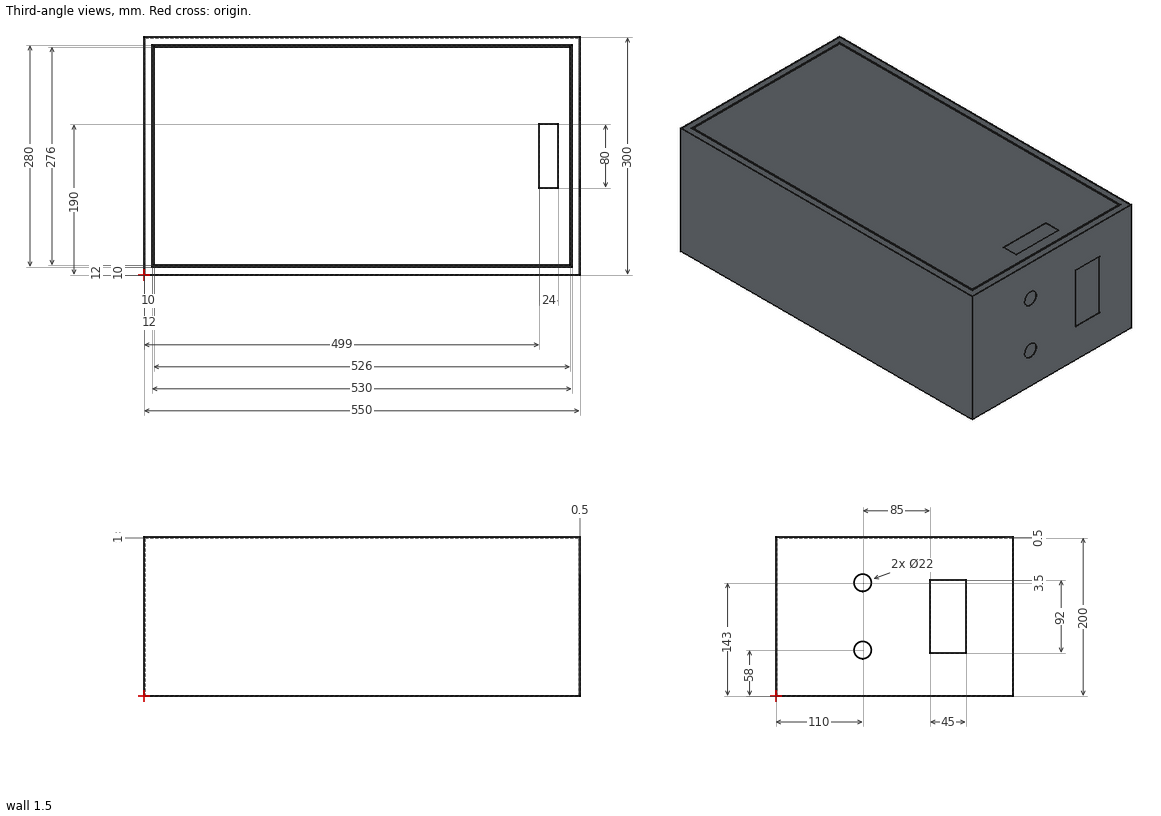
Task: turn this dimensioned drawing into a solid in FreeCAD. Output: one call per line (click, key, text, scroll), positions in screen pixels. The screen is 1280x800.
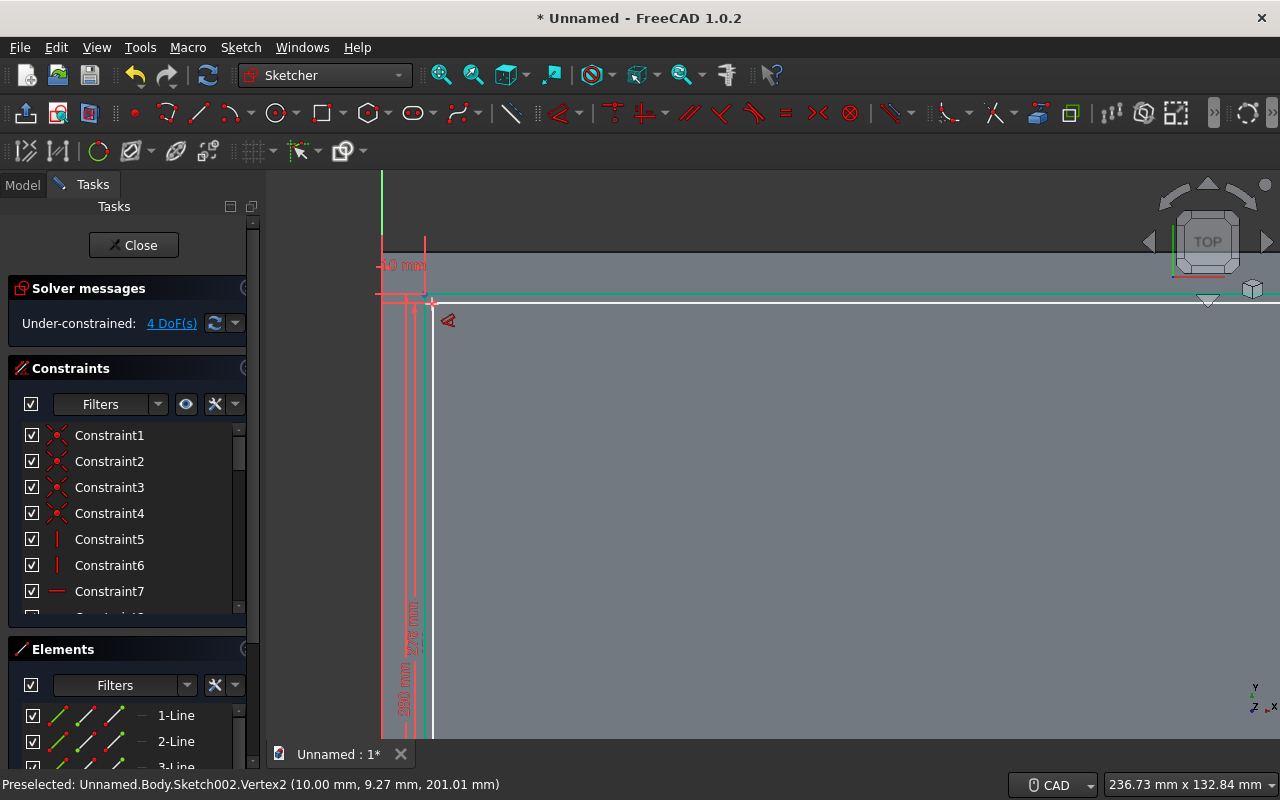
click(433, 303)
click(408, 245)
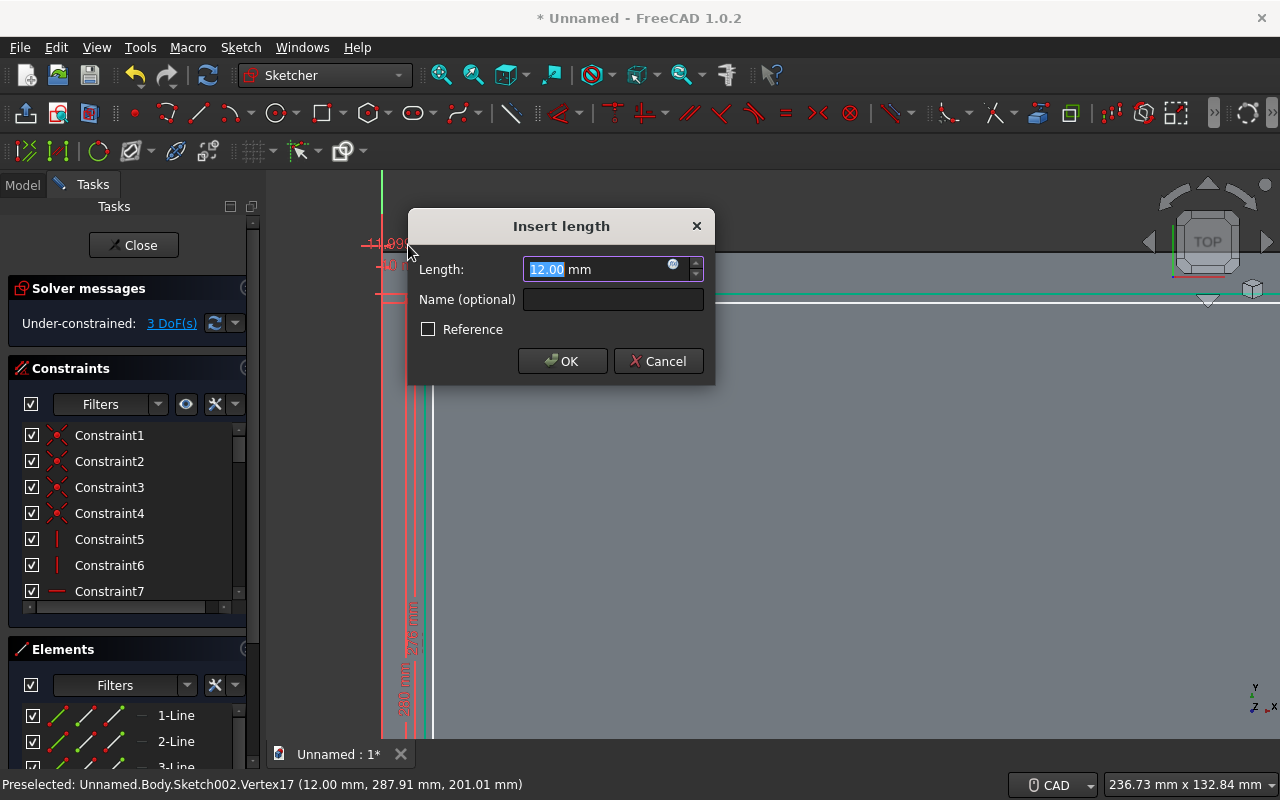
text(12)
key(Return)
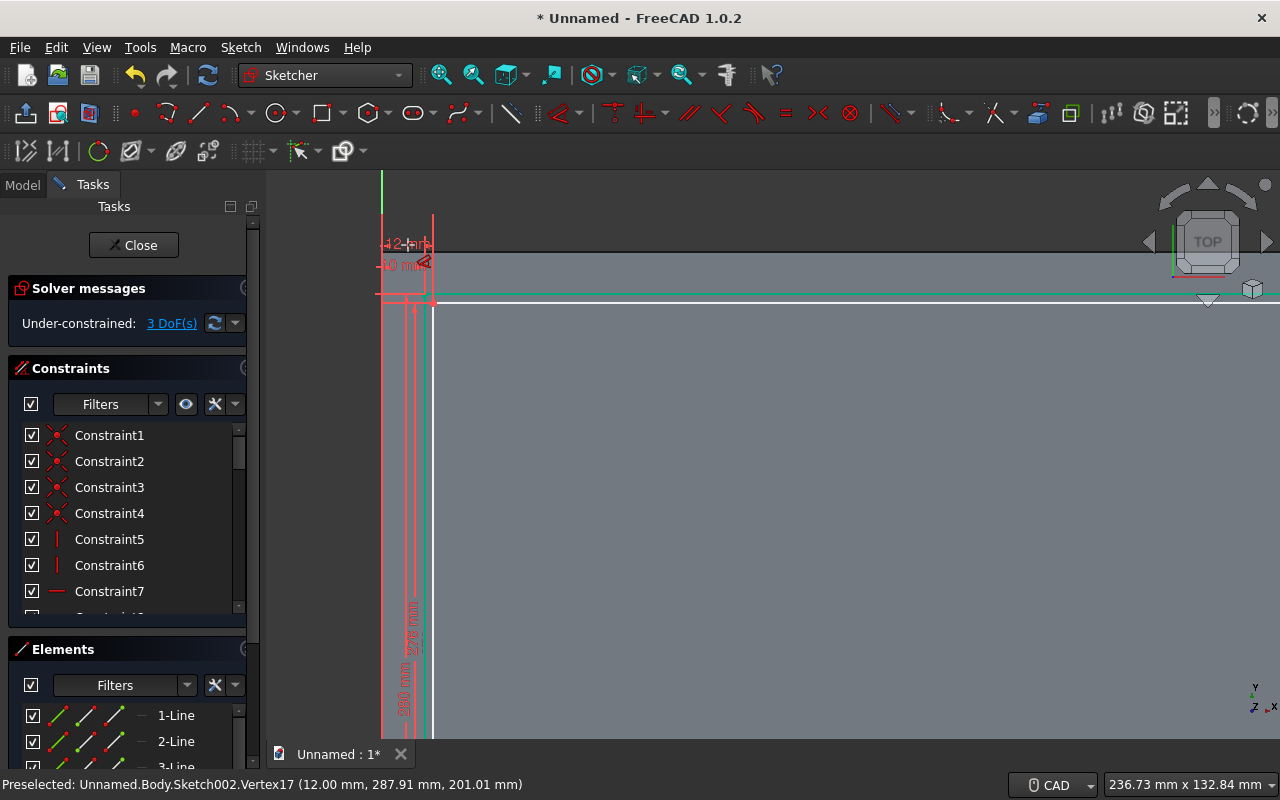
scroll(432, 304, down, 7)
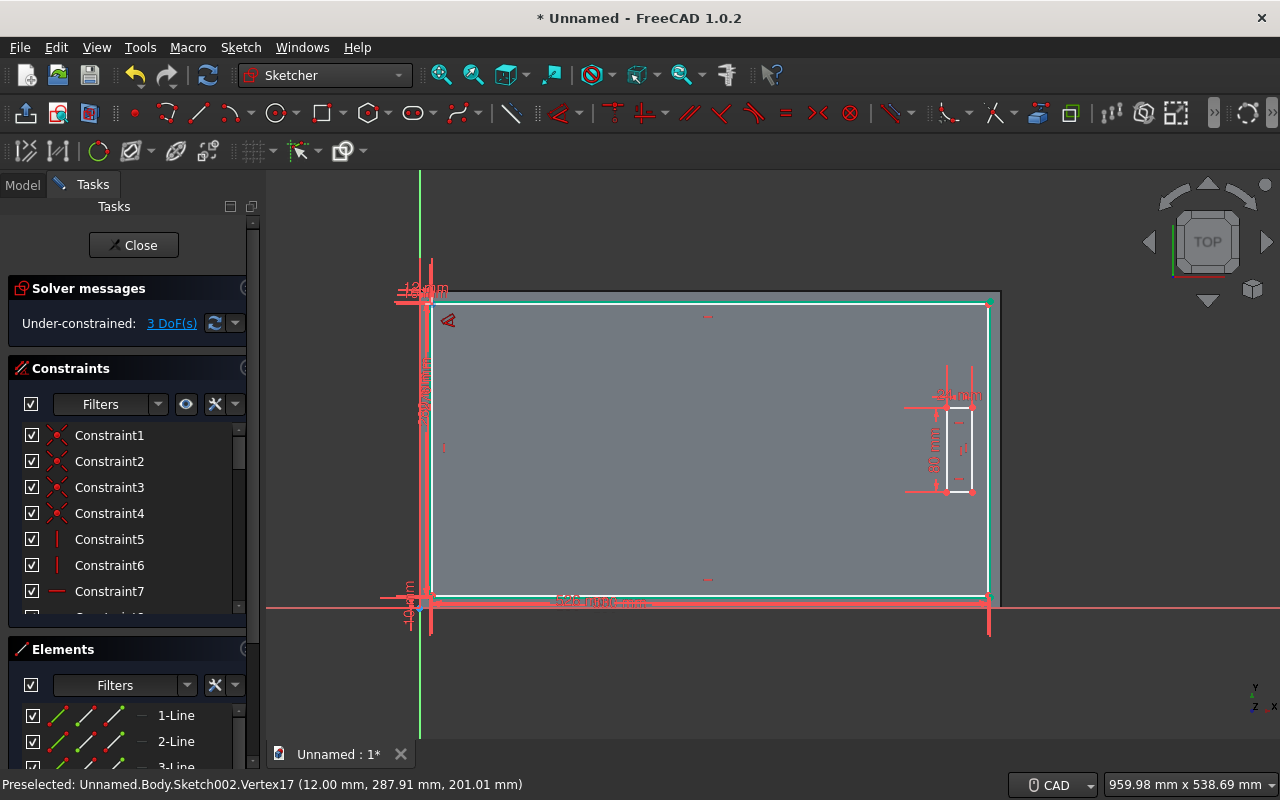
scroll(432, 596, up, 8)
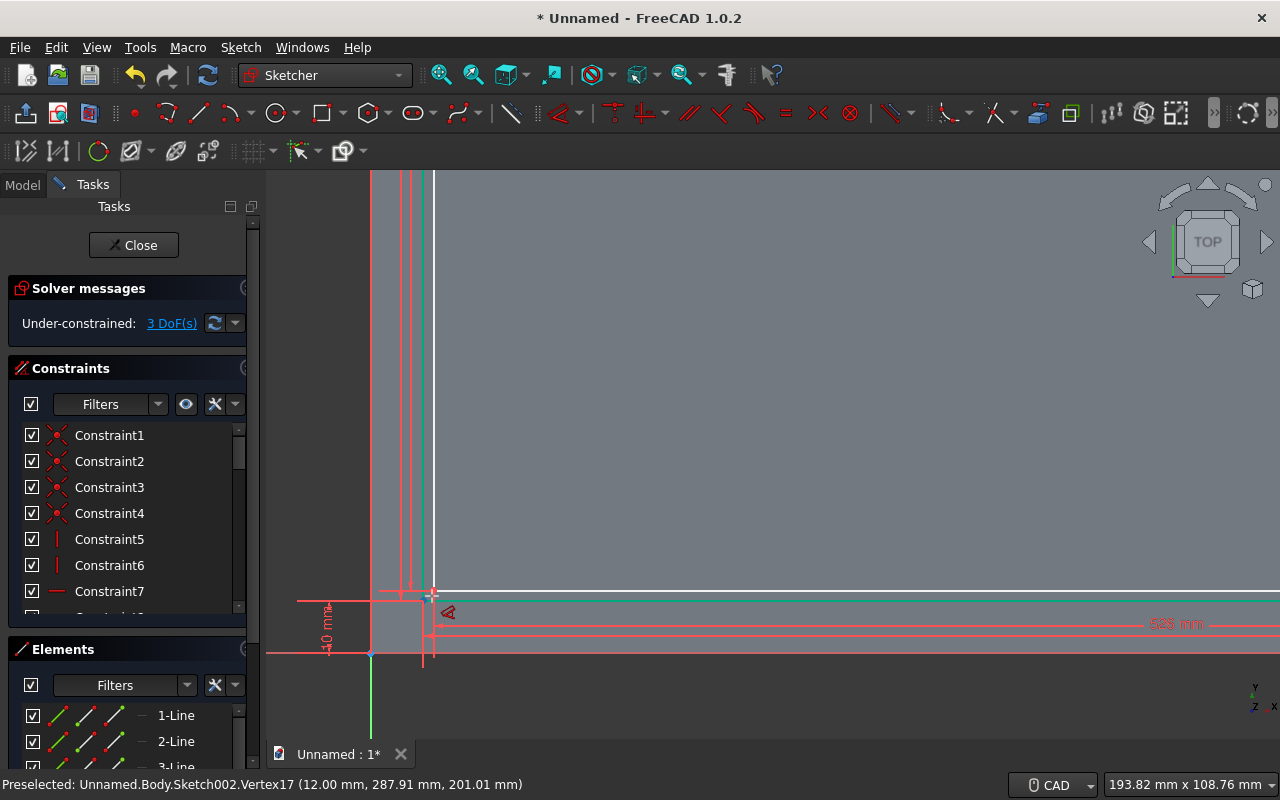
click(434, 591)
click(337, 608)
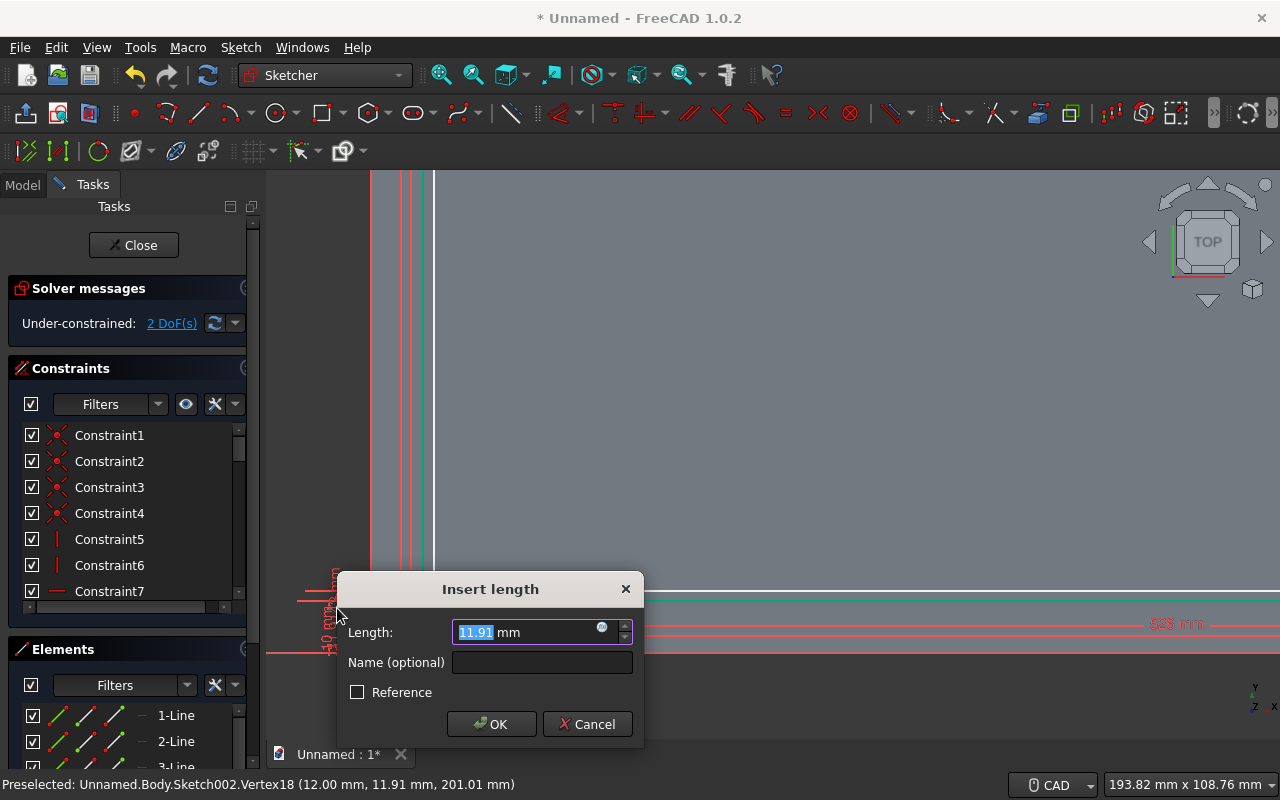
text(12)
key(Return)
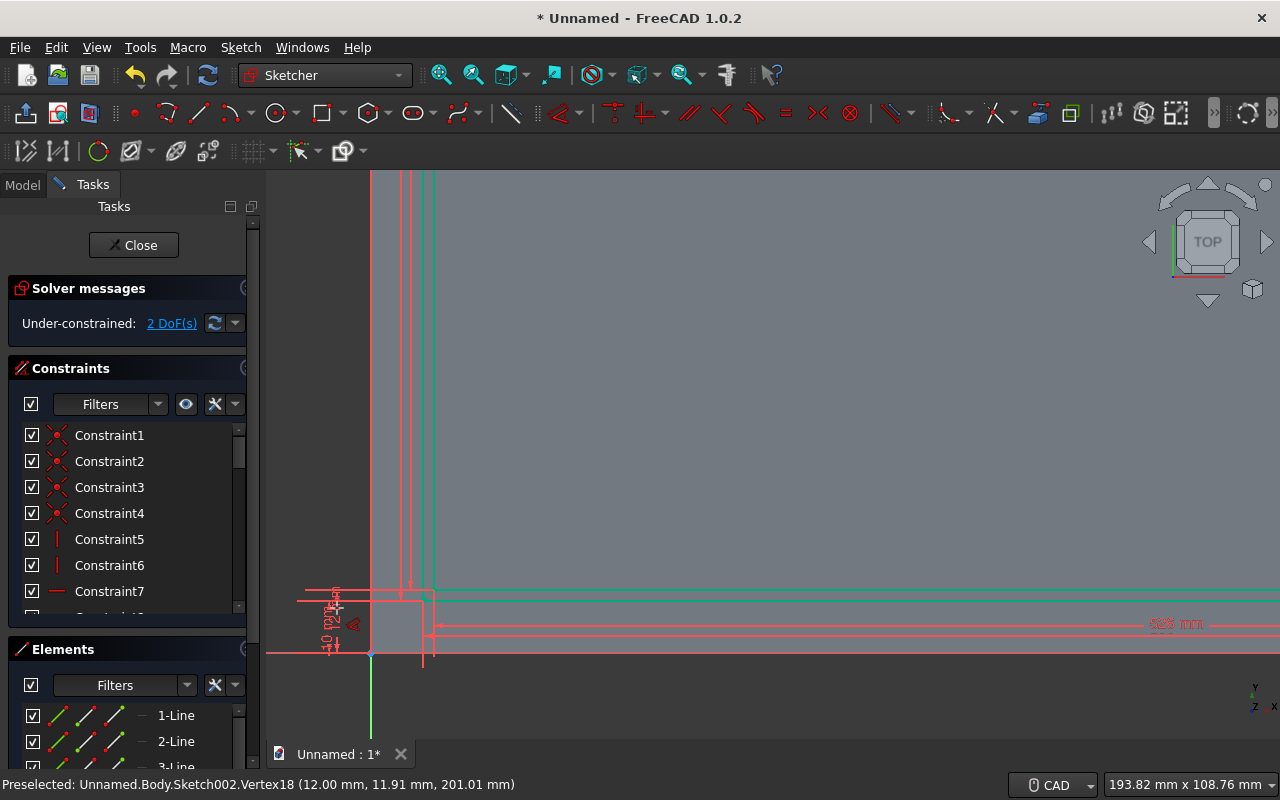
scroll(432, 596, down, 8)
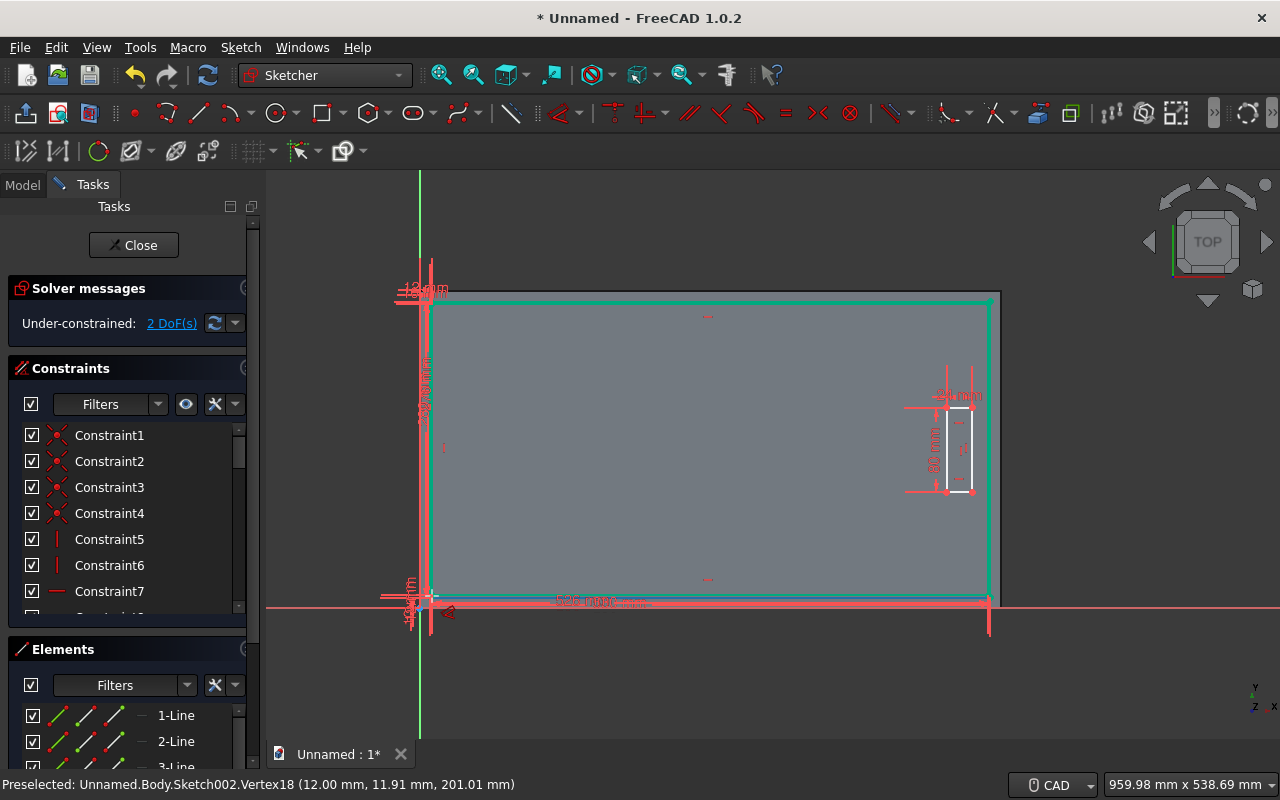
click(947, 408)
click(683, 642)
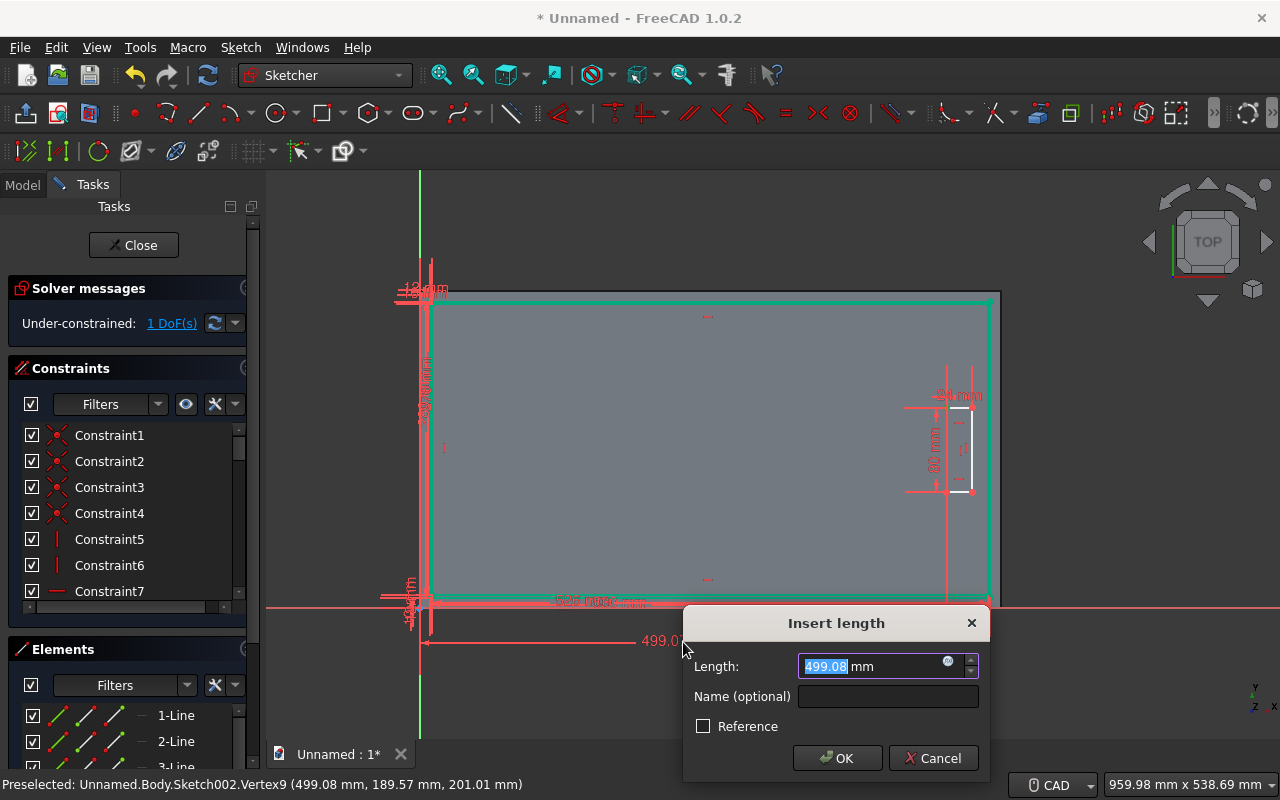
text(499)
key(Return)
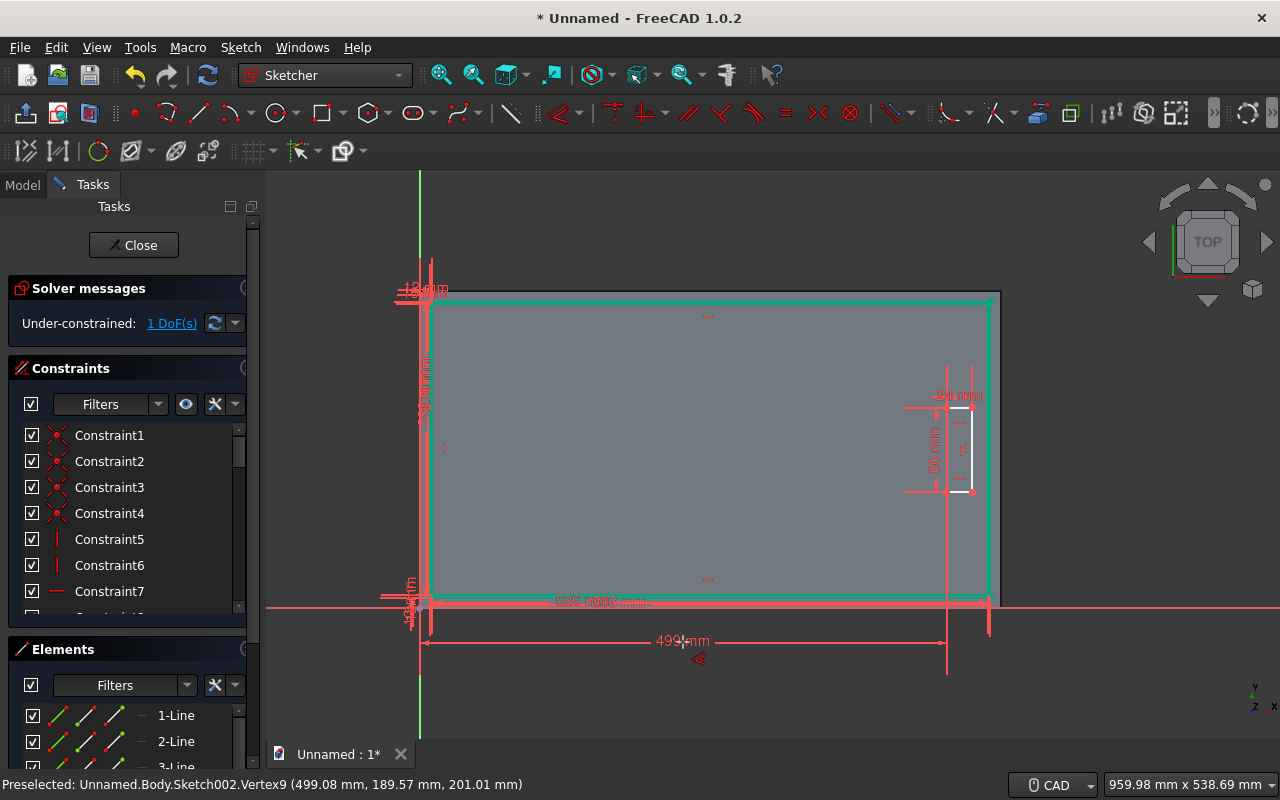
click(947, 408)
click(386, 508)